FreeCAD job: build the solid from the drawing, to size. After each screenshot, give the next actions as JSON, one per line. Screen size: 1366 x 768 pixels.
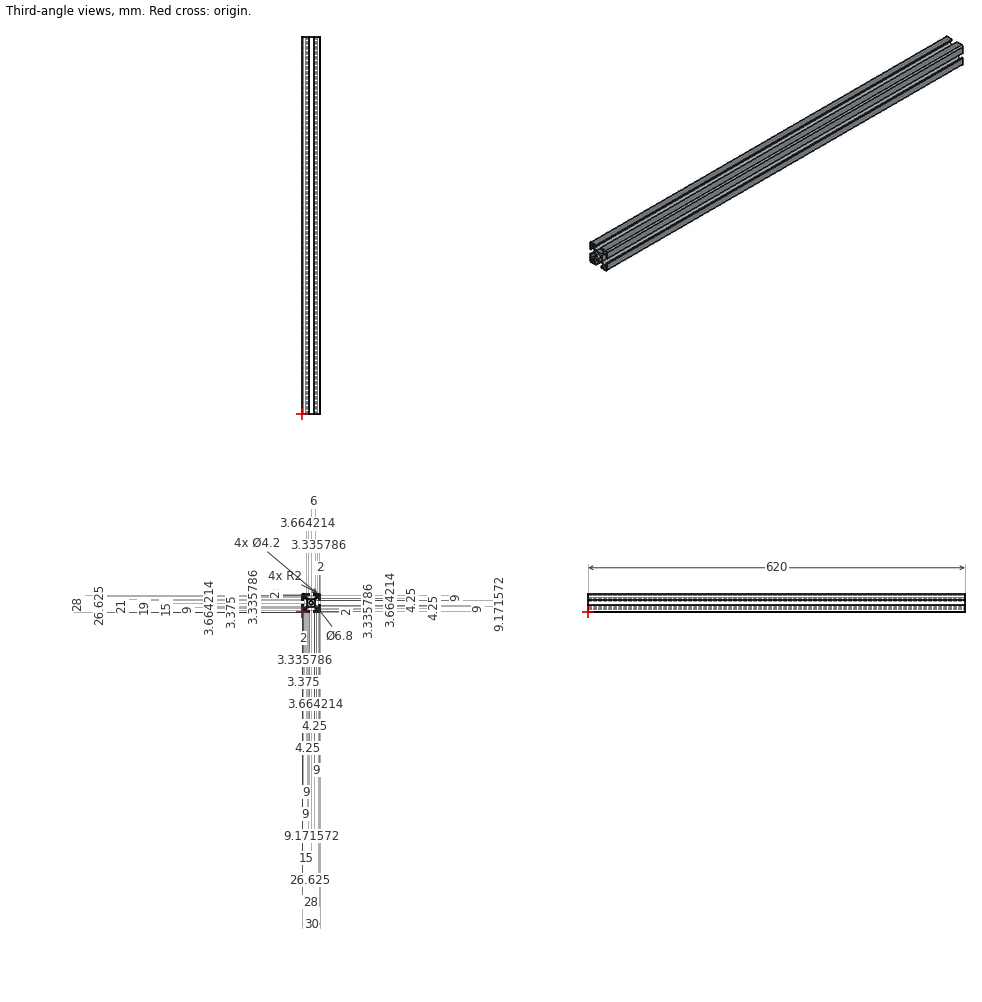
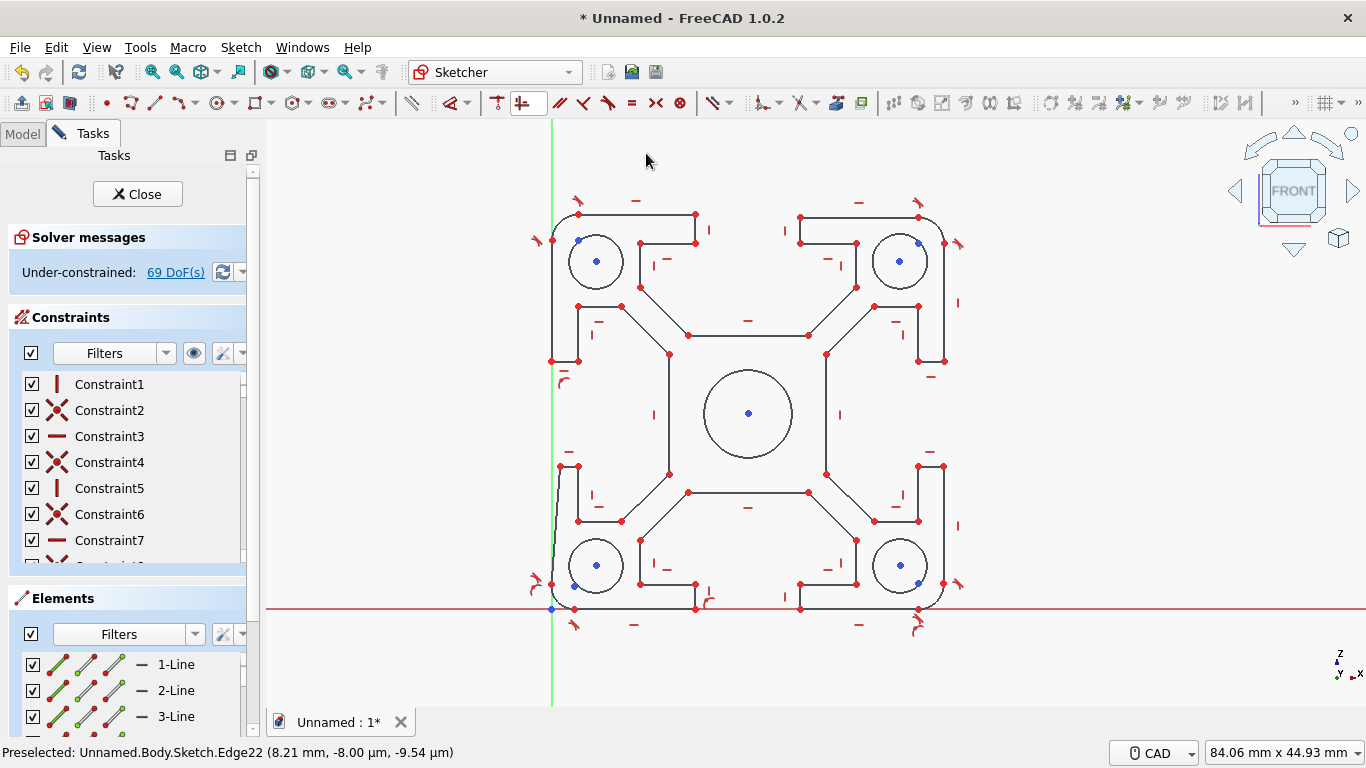
{"action": "left_click", "coordinate": [554, 549]}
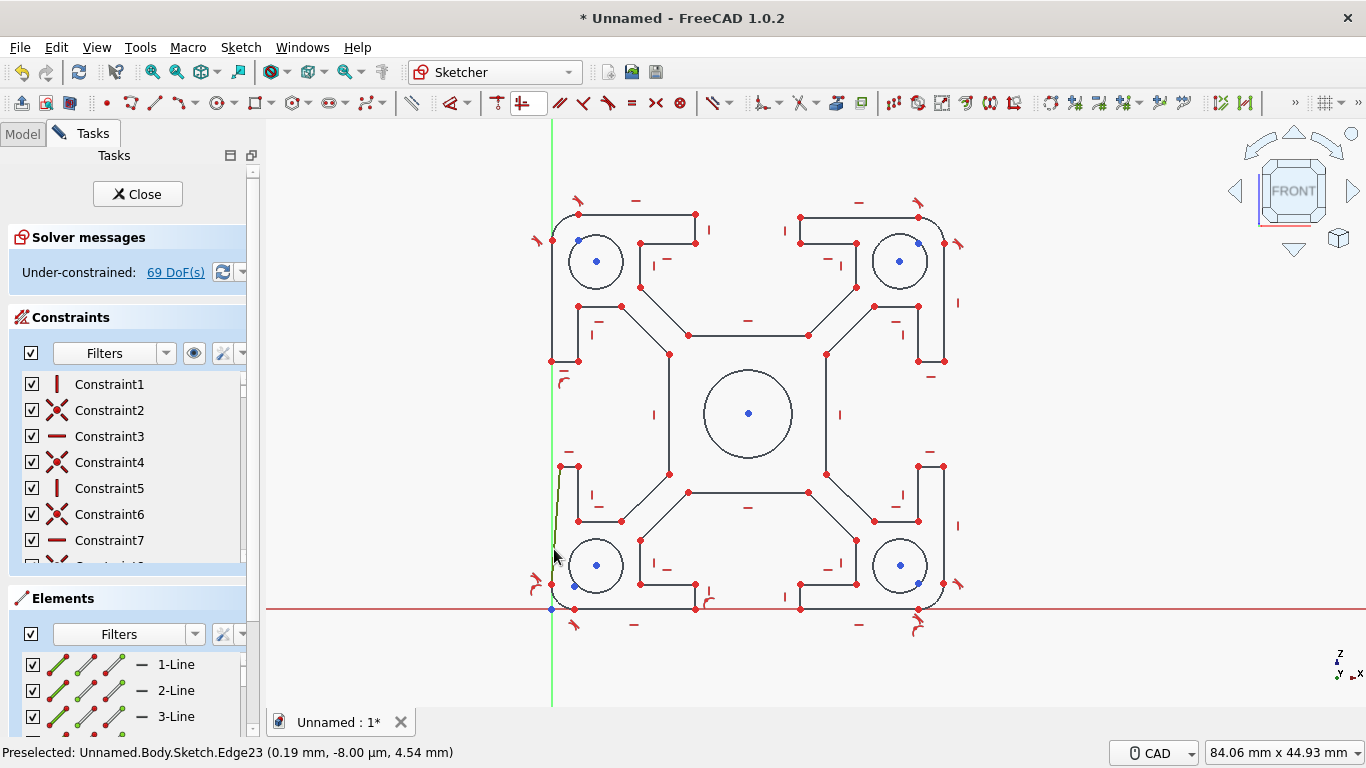
{"action": "key", "text": "v"}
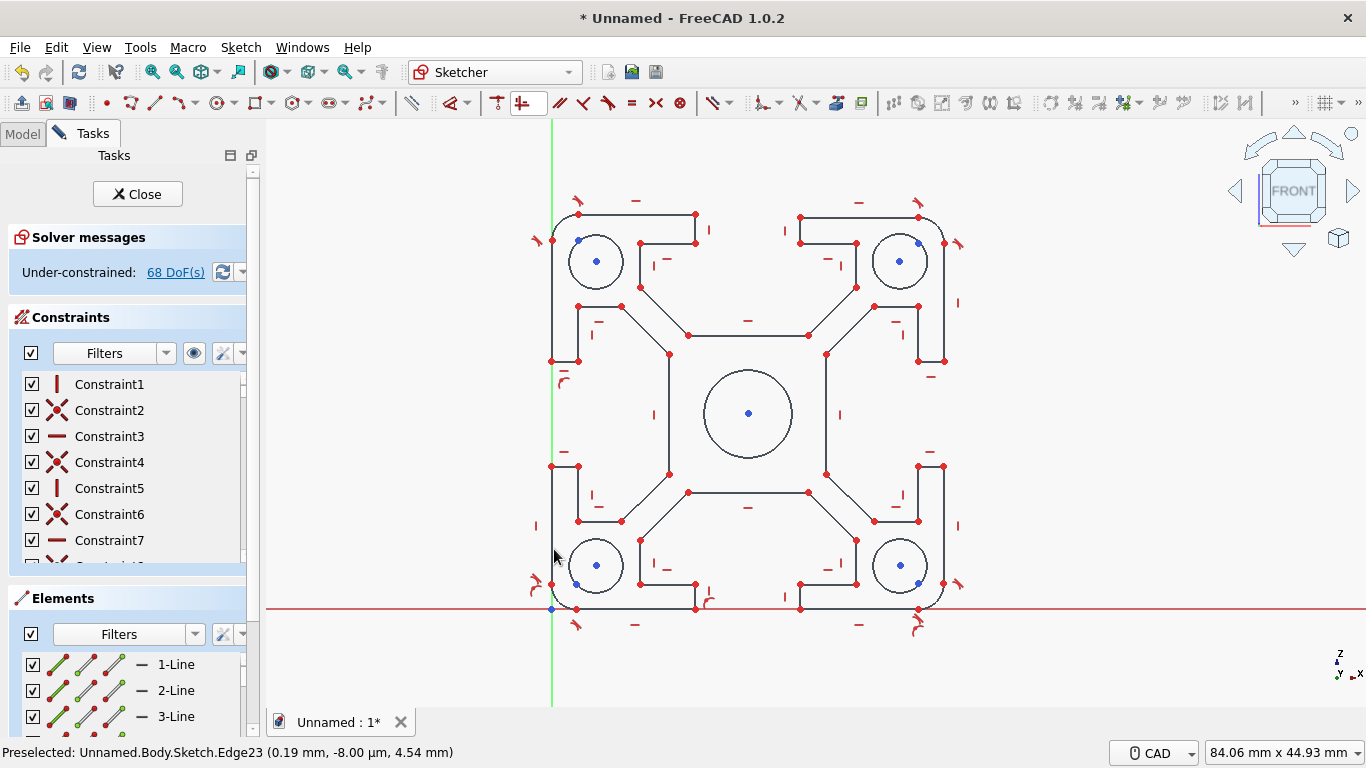
{"action": "left_click", "coordinate": [552, 325]}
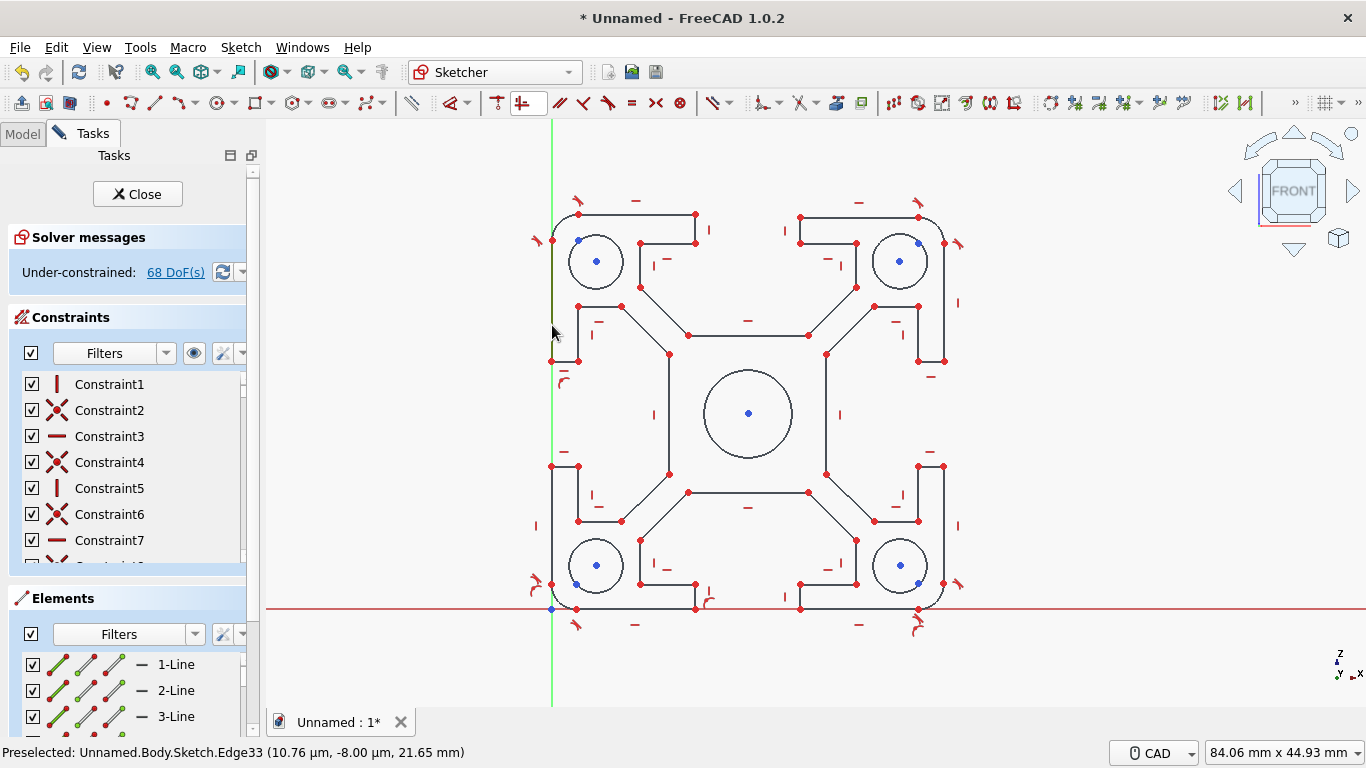
{"action": "key", "text": "v"}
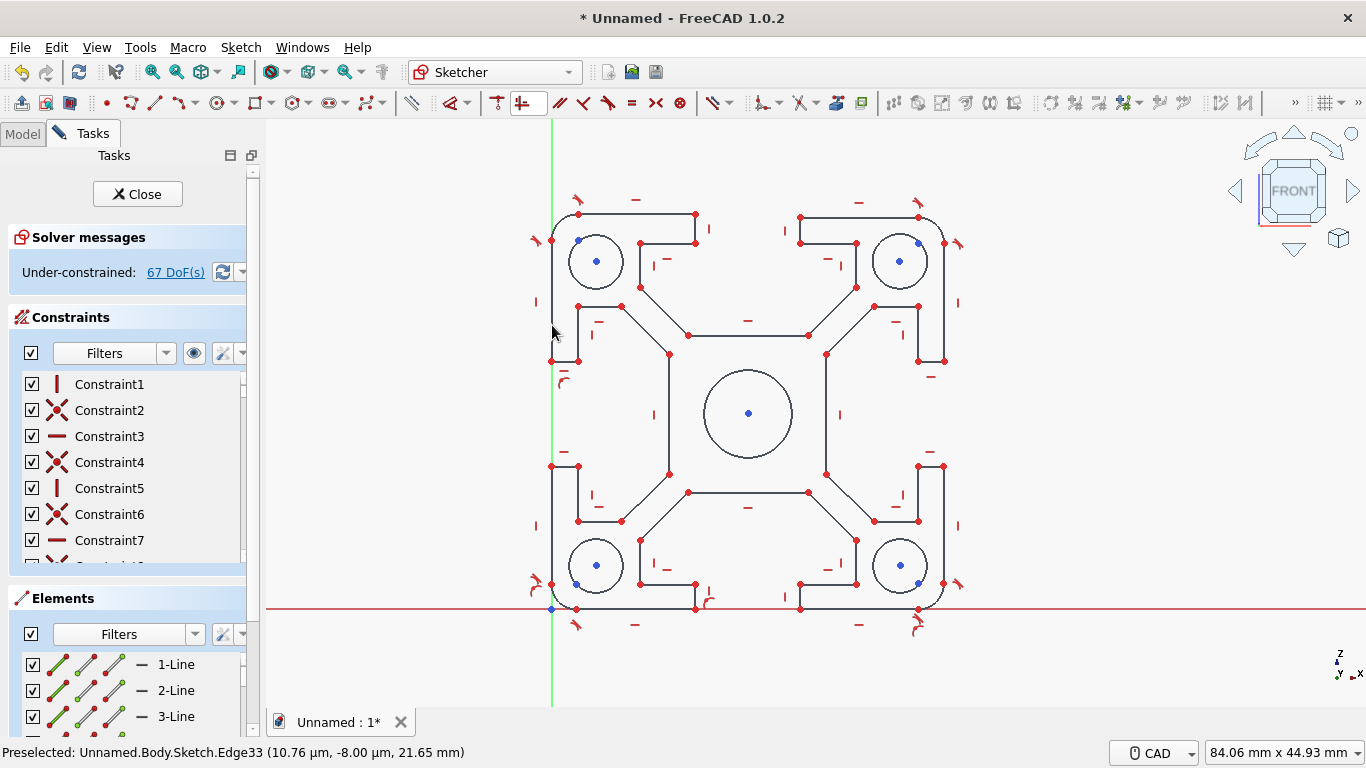
{"action": "left_click", "coordinate": [930, 607]}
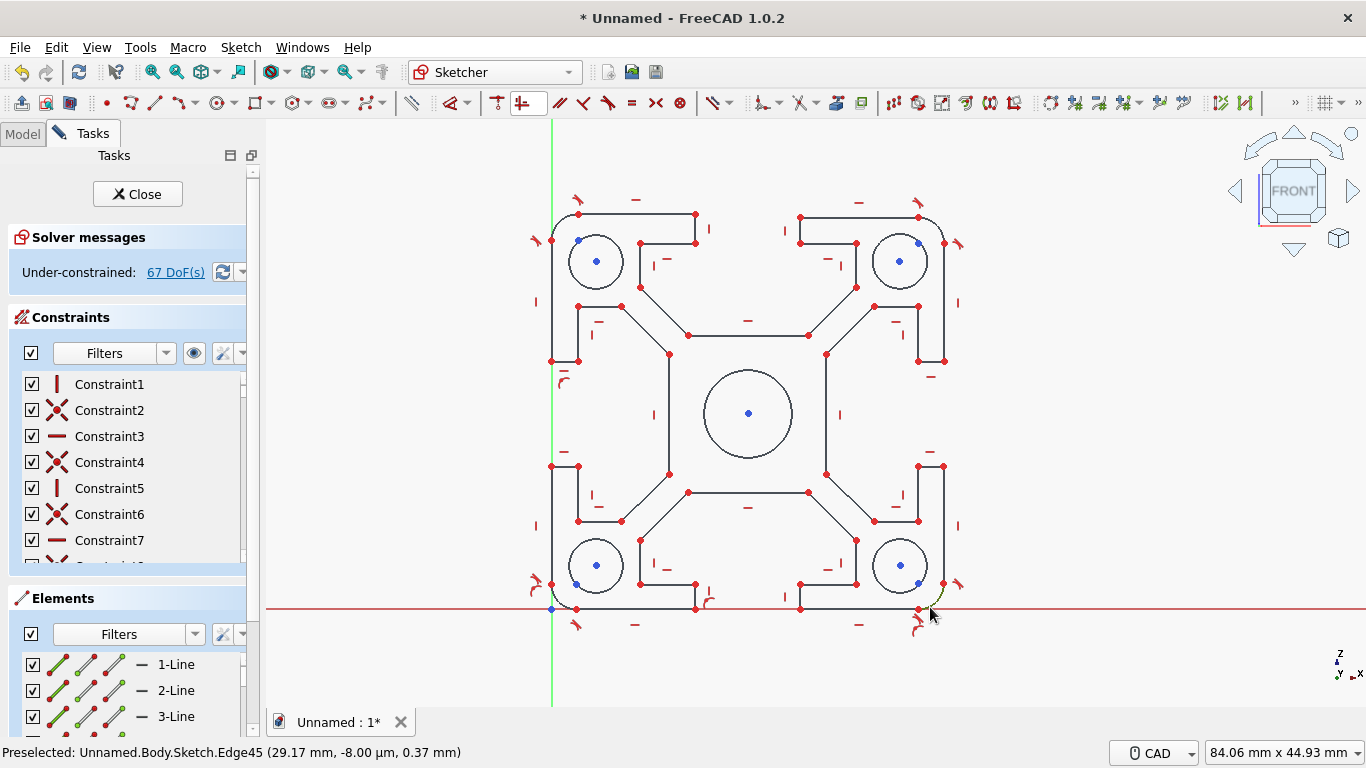
{"action": "left_click", "coordinate": [554, 596]}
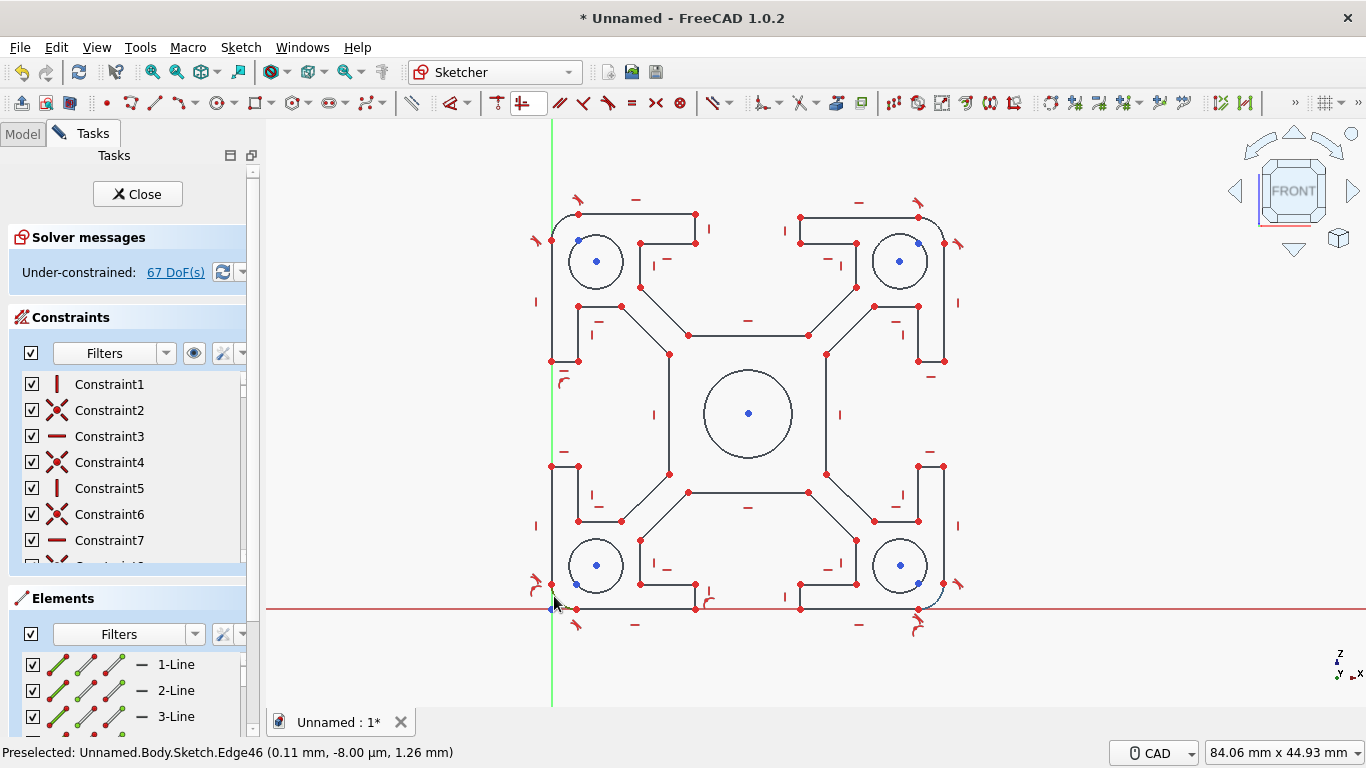
{"action": "left_click", "coordinate": [566, 217]}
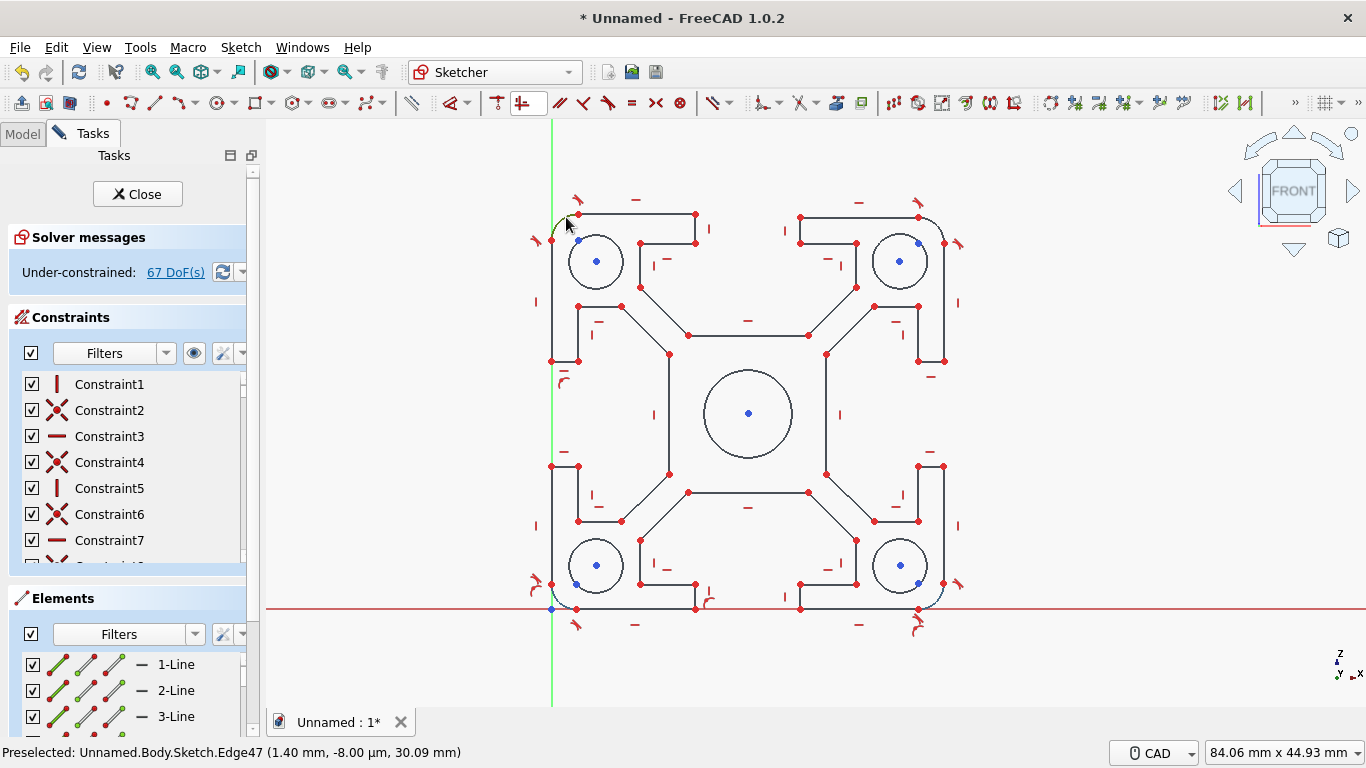
{"action": "left_click", "coordinate": [941, 232]}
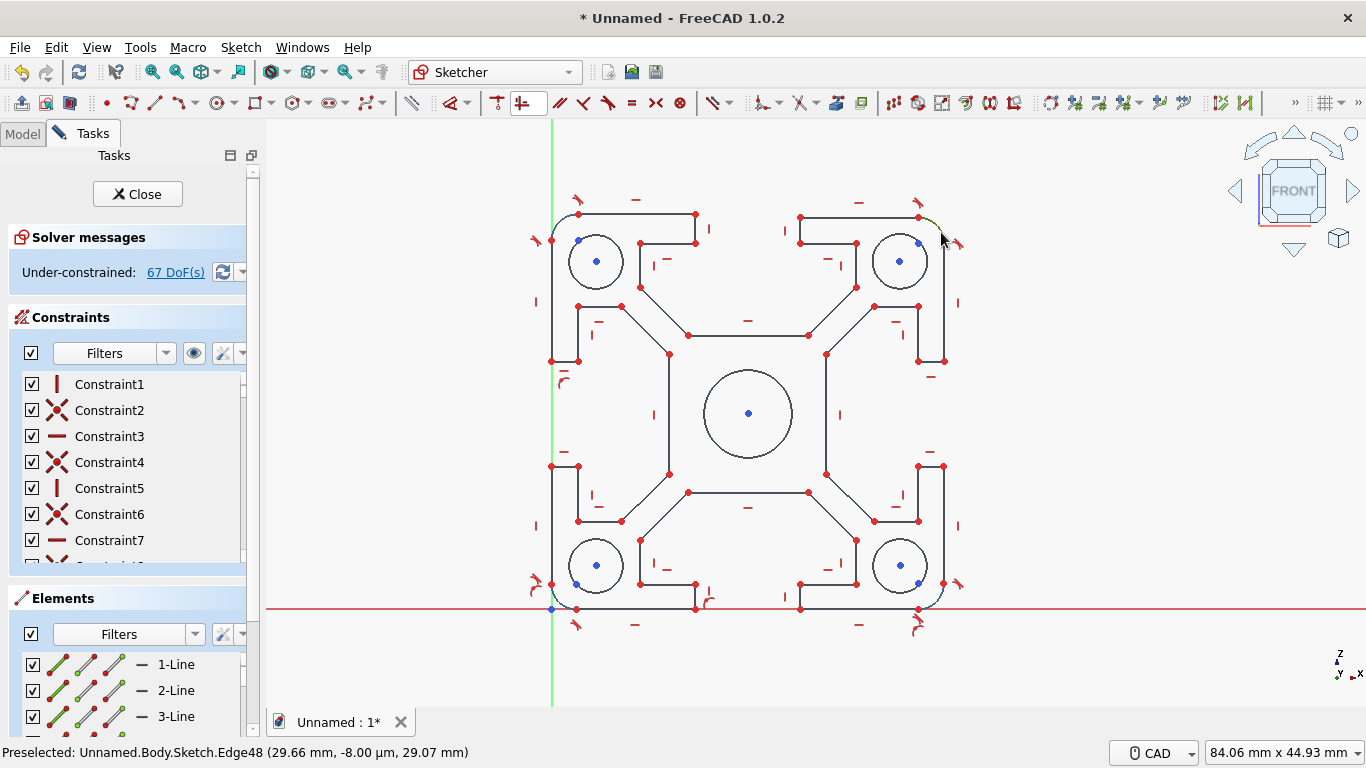
{"action": "key", "text": "e"}